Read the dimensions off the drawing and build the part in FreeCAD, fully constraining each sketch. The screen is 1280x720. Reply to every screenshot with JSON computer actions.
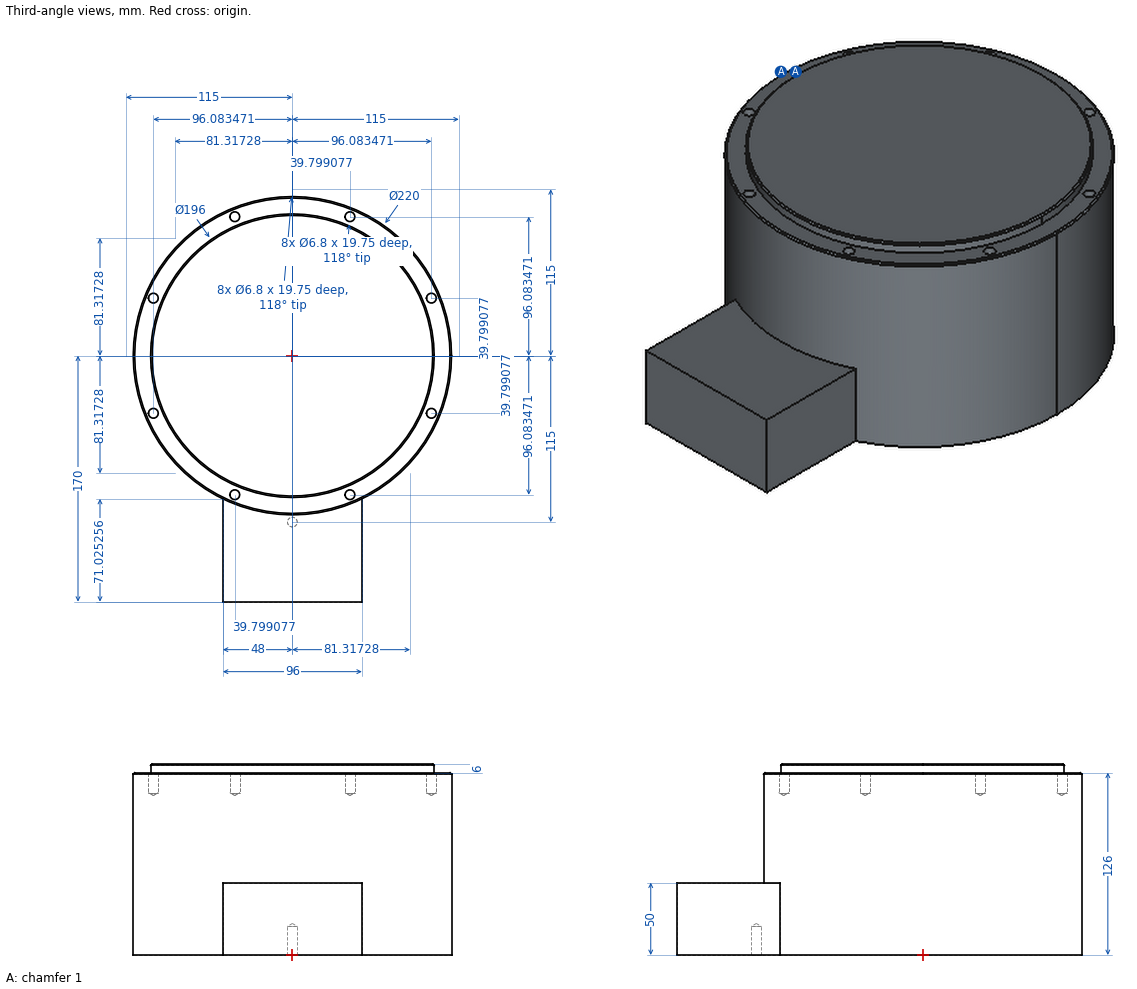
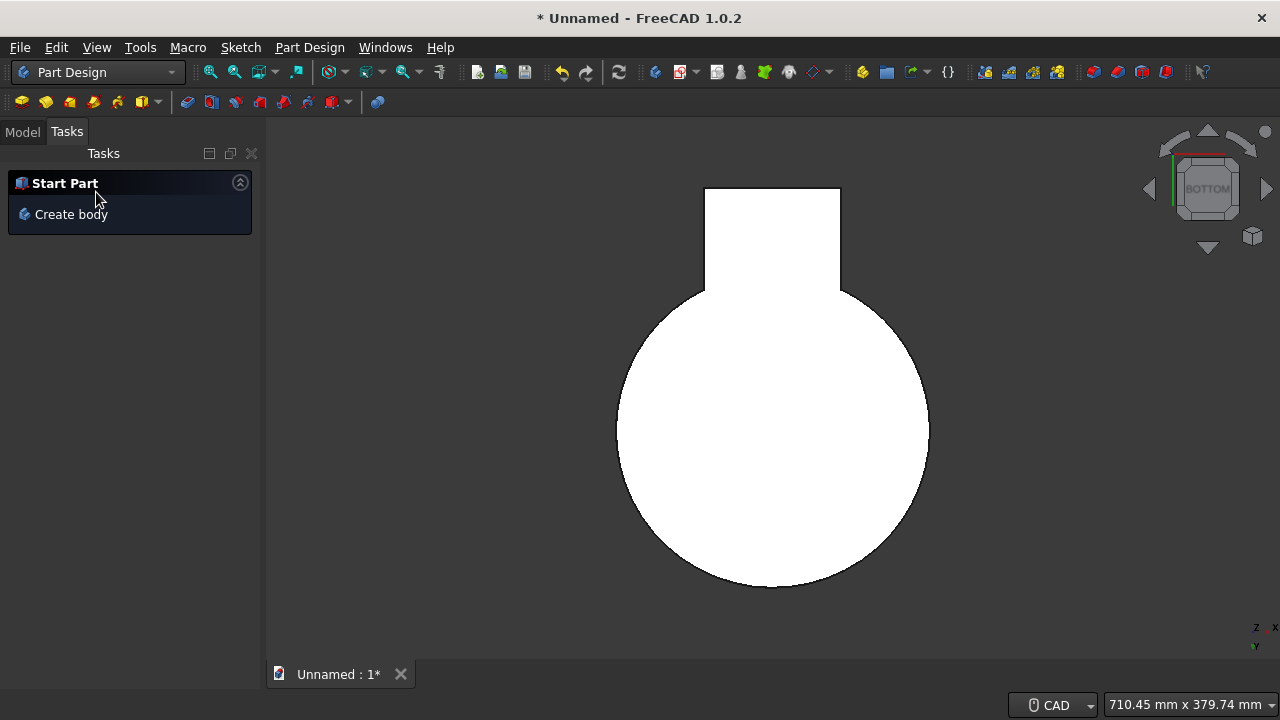
{"action": "left_click", "coordinate": [773, 444]}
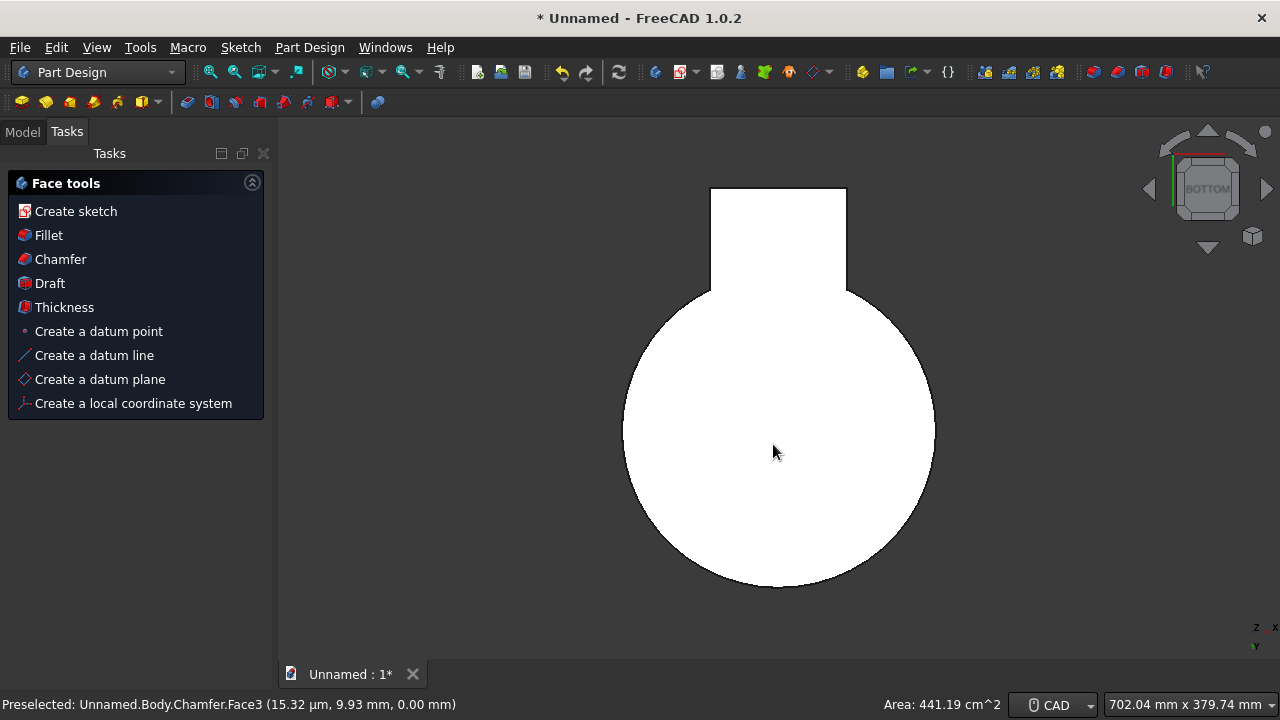
{"action": "left_click", "coordinate": [680, 72]}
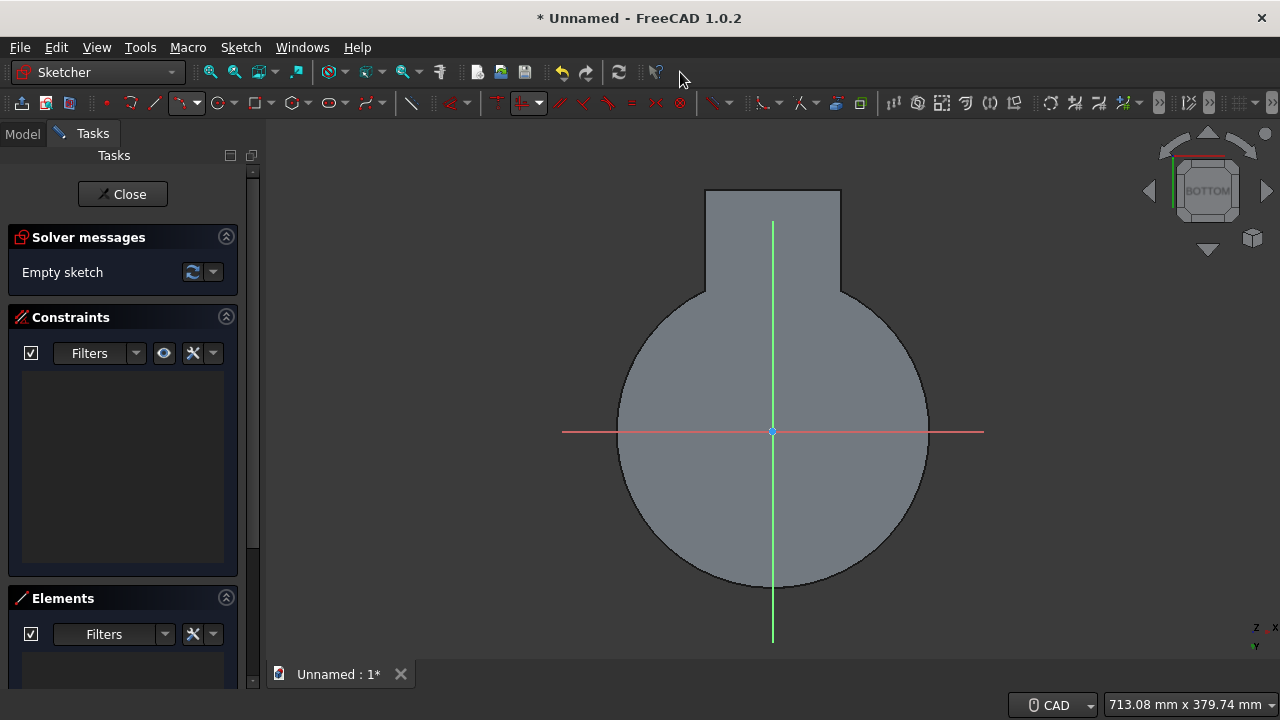
{"action": "left_click", "coordinate": [218, 104]}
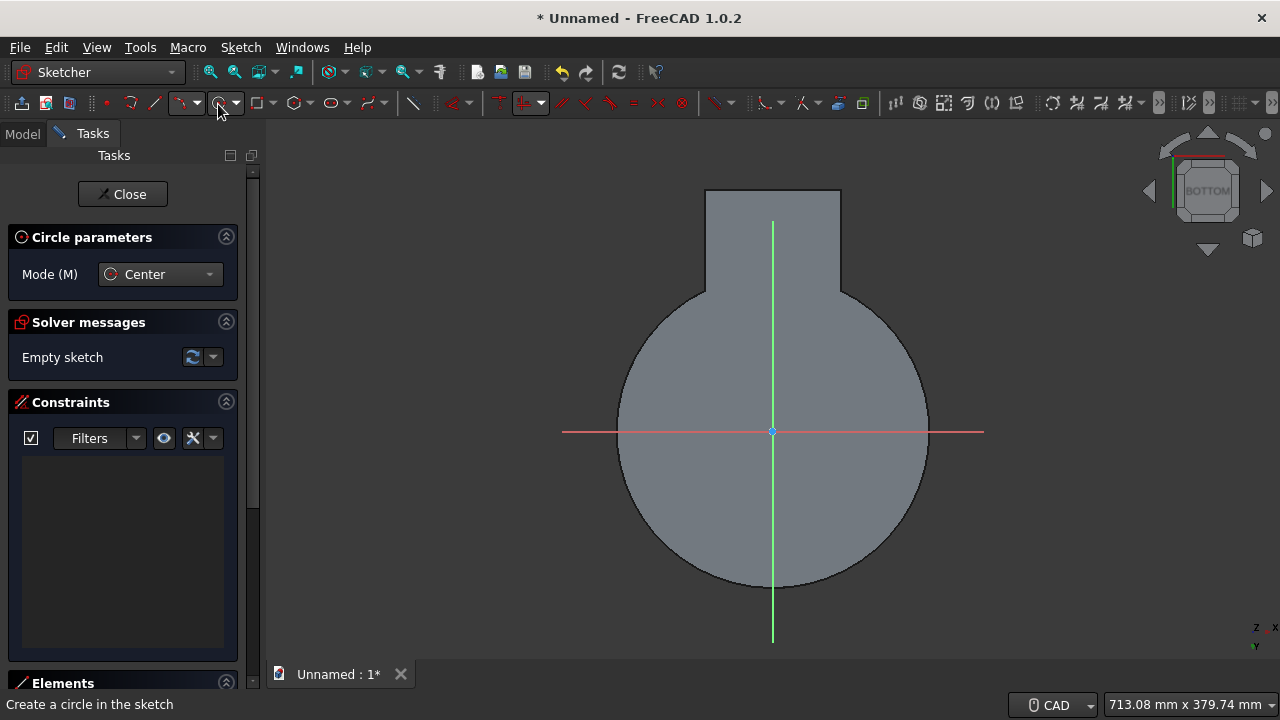
{"action": "scroll", "coordinate": [773, 595], "scroll_direction": "up", "scroll_amount": 8}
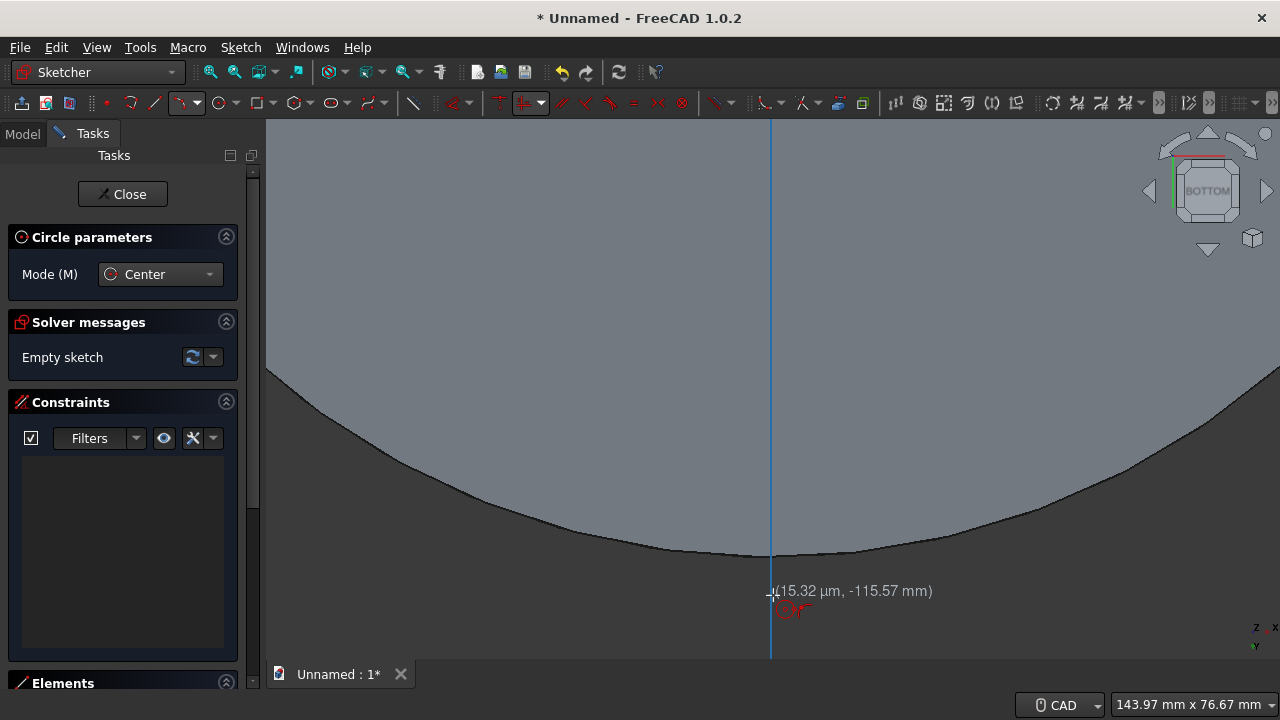
{"action": "scroll", "coordinate": [688, 542], "scroll_direction": "down", "scroll_amount": 8}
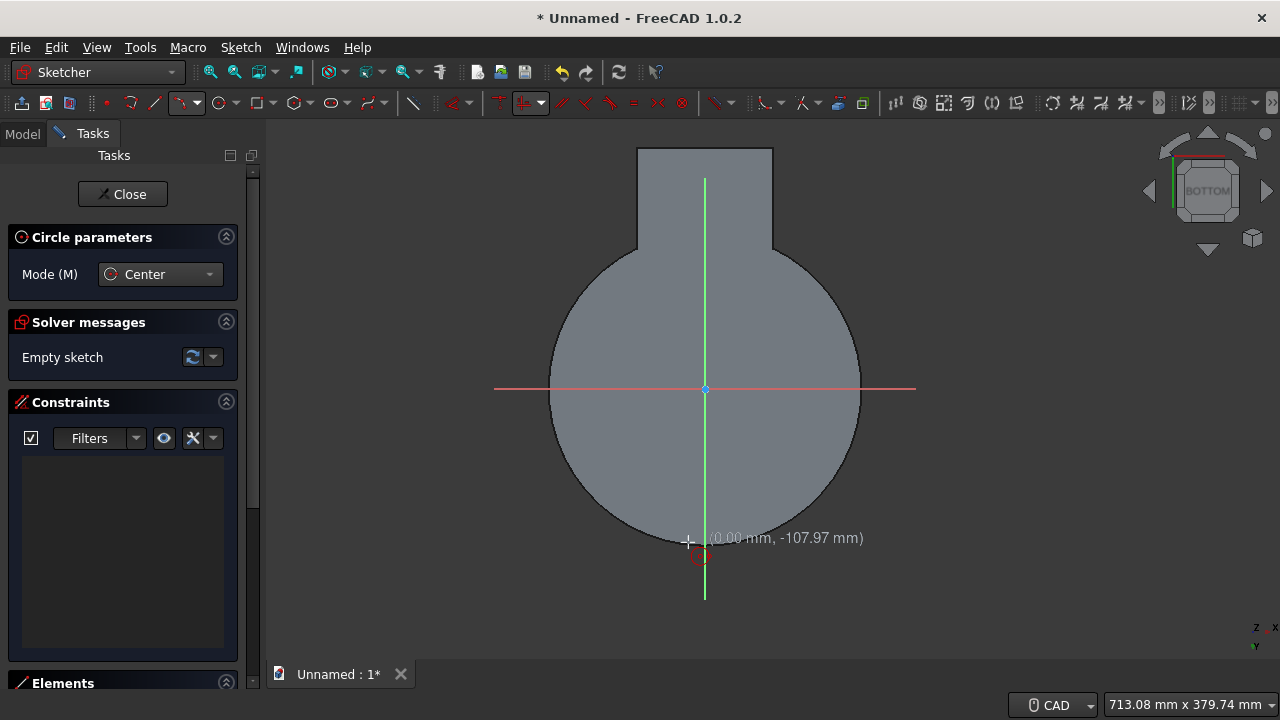
{"action": "left_click", "coordinate": [705, 553]}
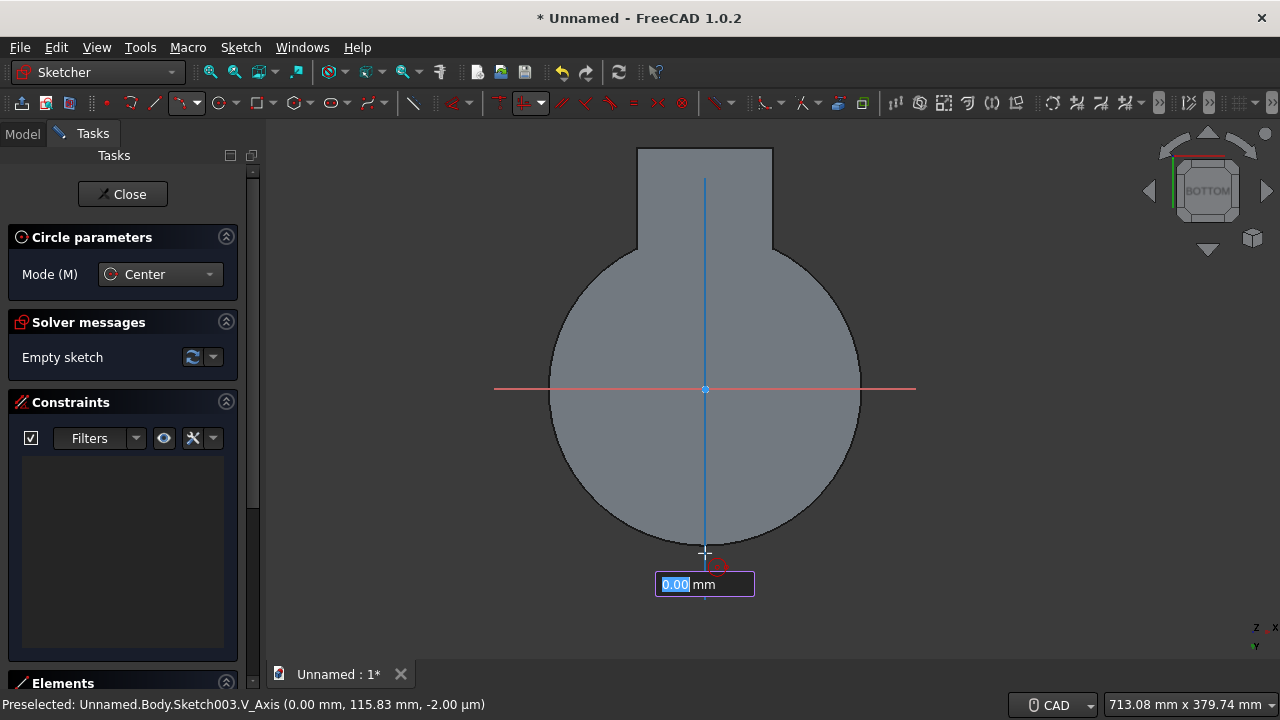
{"action": "scroll", "coordinate": [710, 551], "scroll_direction": "up", "scroll_amount": 7}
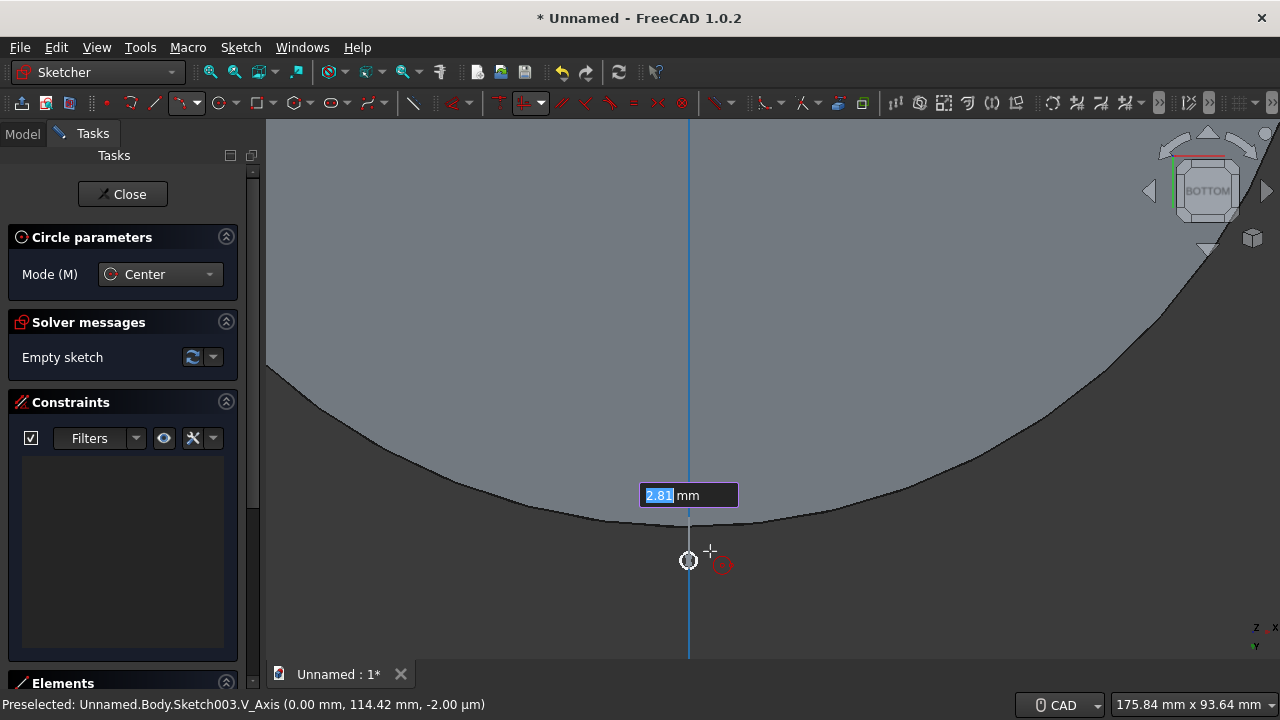
{"action": "left_click", "coordinate": [707, 549]}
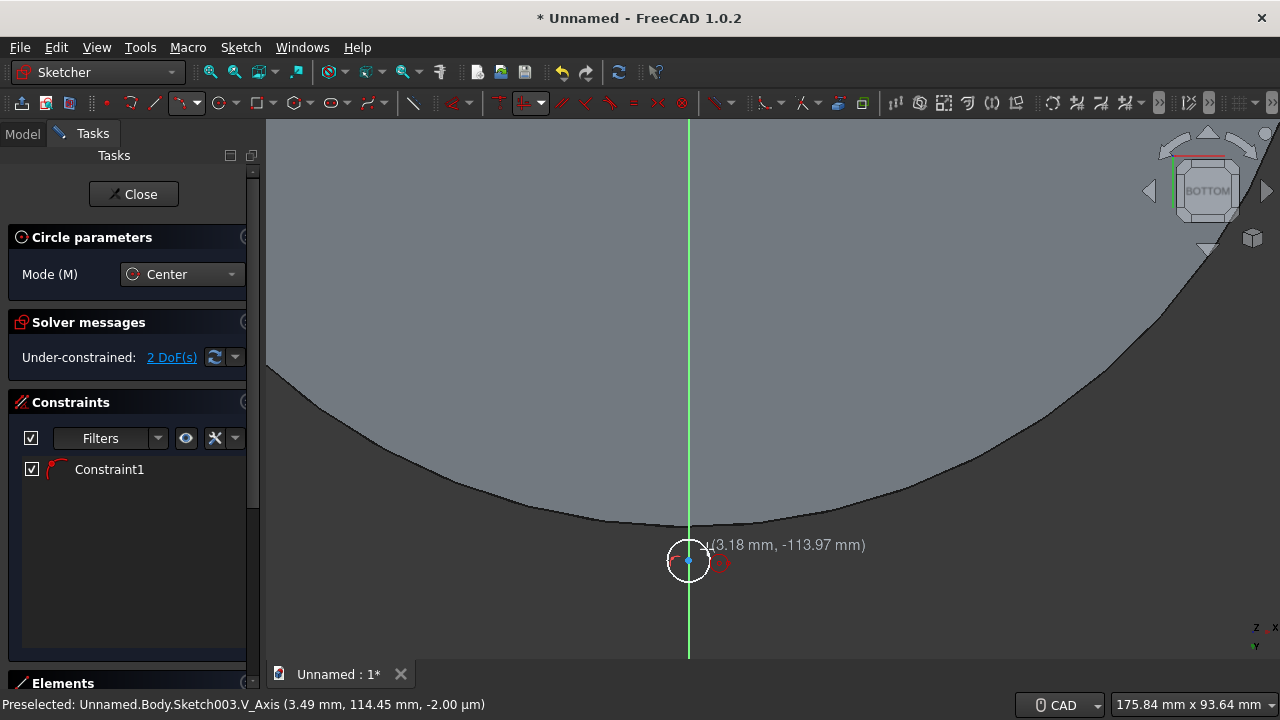
{"action": "scroll", "coordinate": [710, 551], "scroll_direction": "down", "scroll_amount": 7}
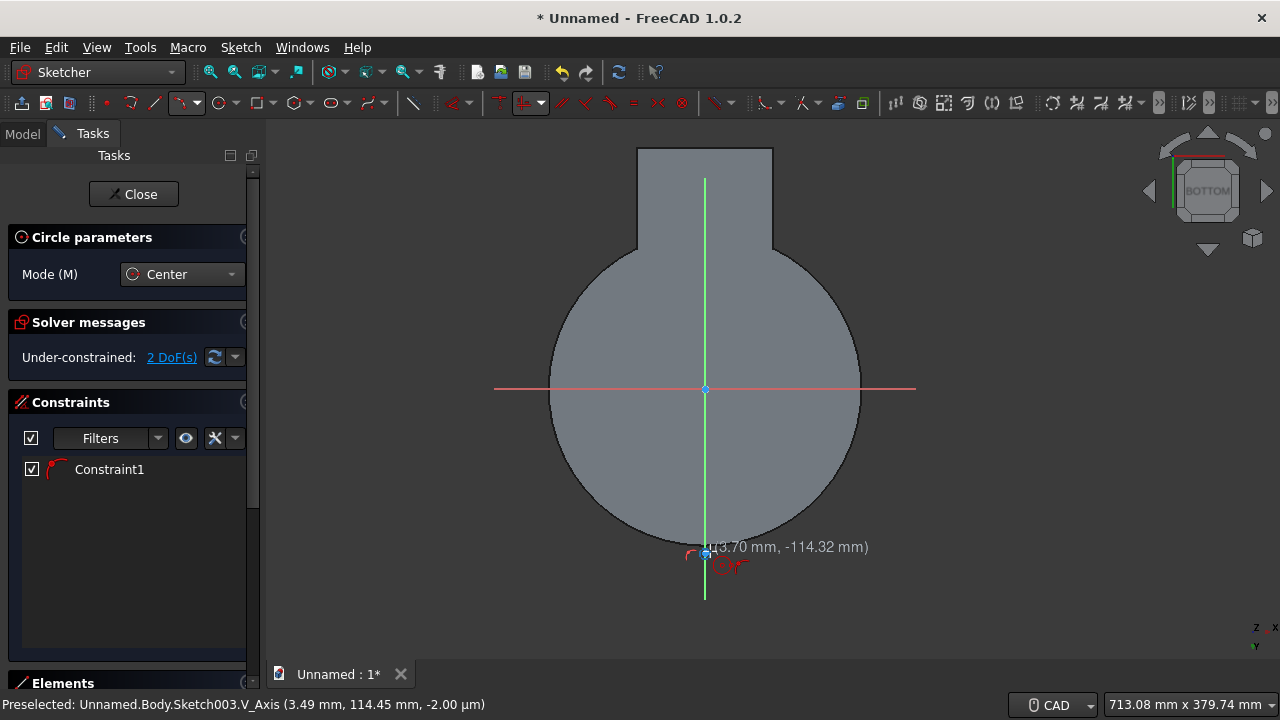
{"action": "scroll", "coordinate": [589, 505], "scroll_direction": "up", "scroll_amount": 8}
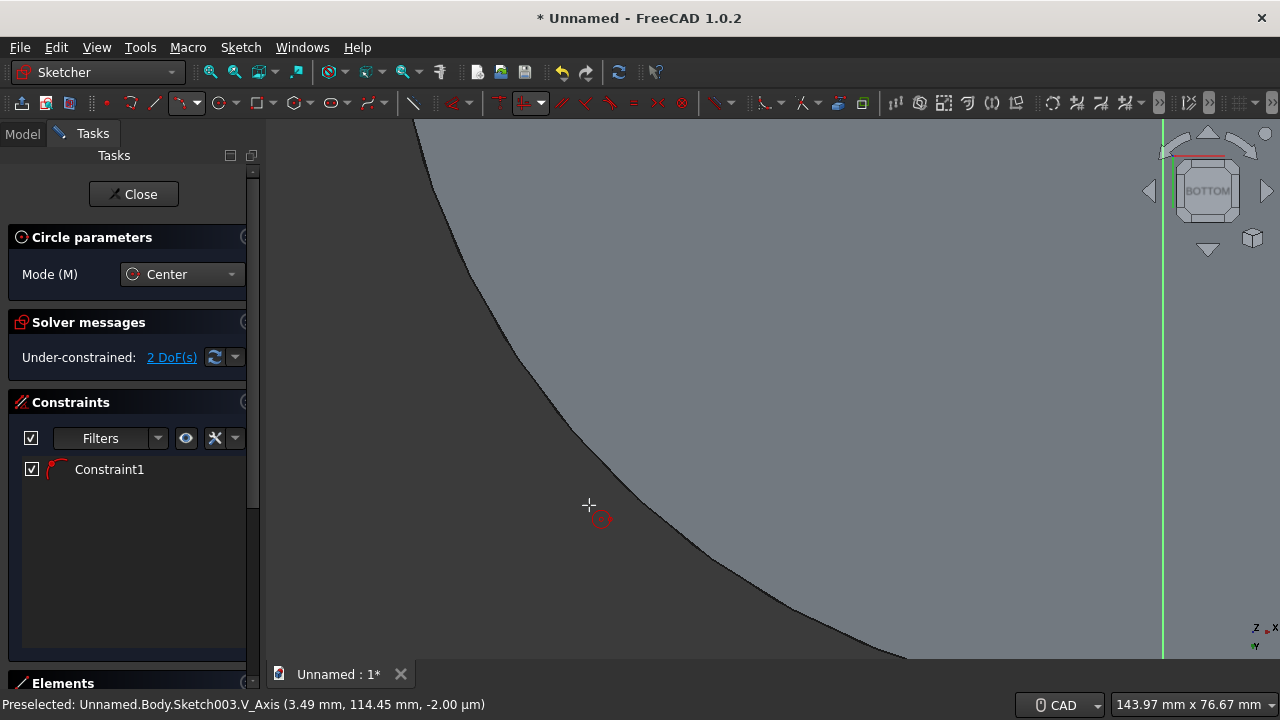
{"action": "scroll", "coordinate": [589, 505], "scroll_direction": "down", "scroll_amount": 8}